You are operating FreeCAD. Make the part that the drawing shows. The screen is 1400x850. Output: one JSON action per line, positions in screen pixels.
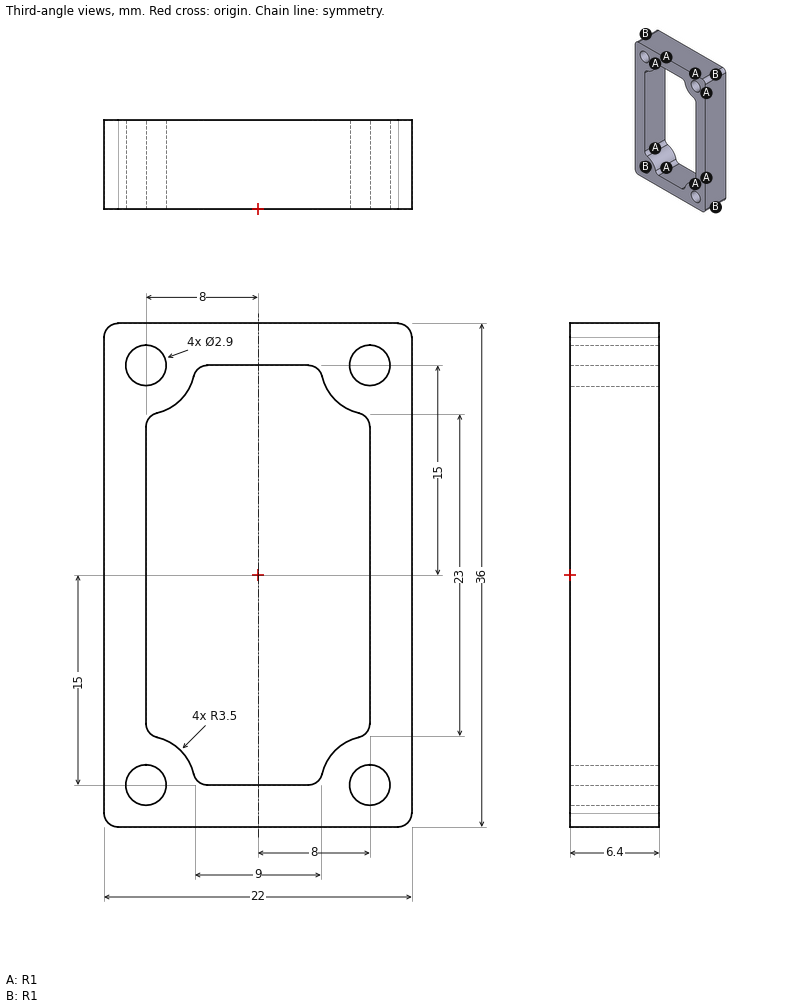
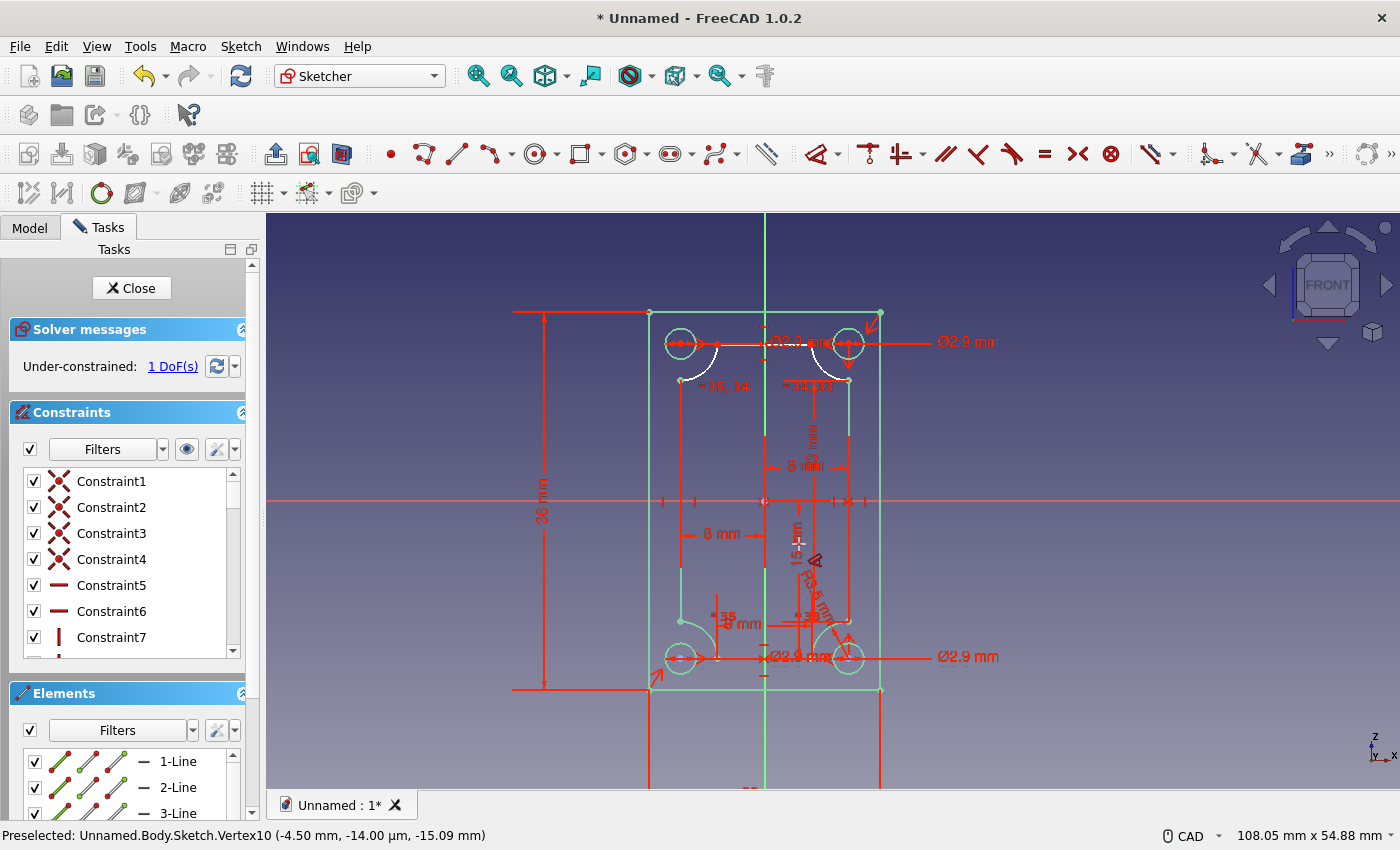
{"action": "left_click", "coordinate": [812, 345]}
{"action": "left_click", "coordinate": [731, 423]}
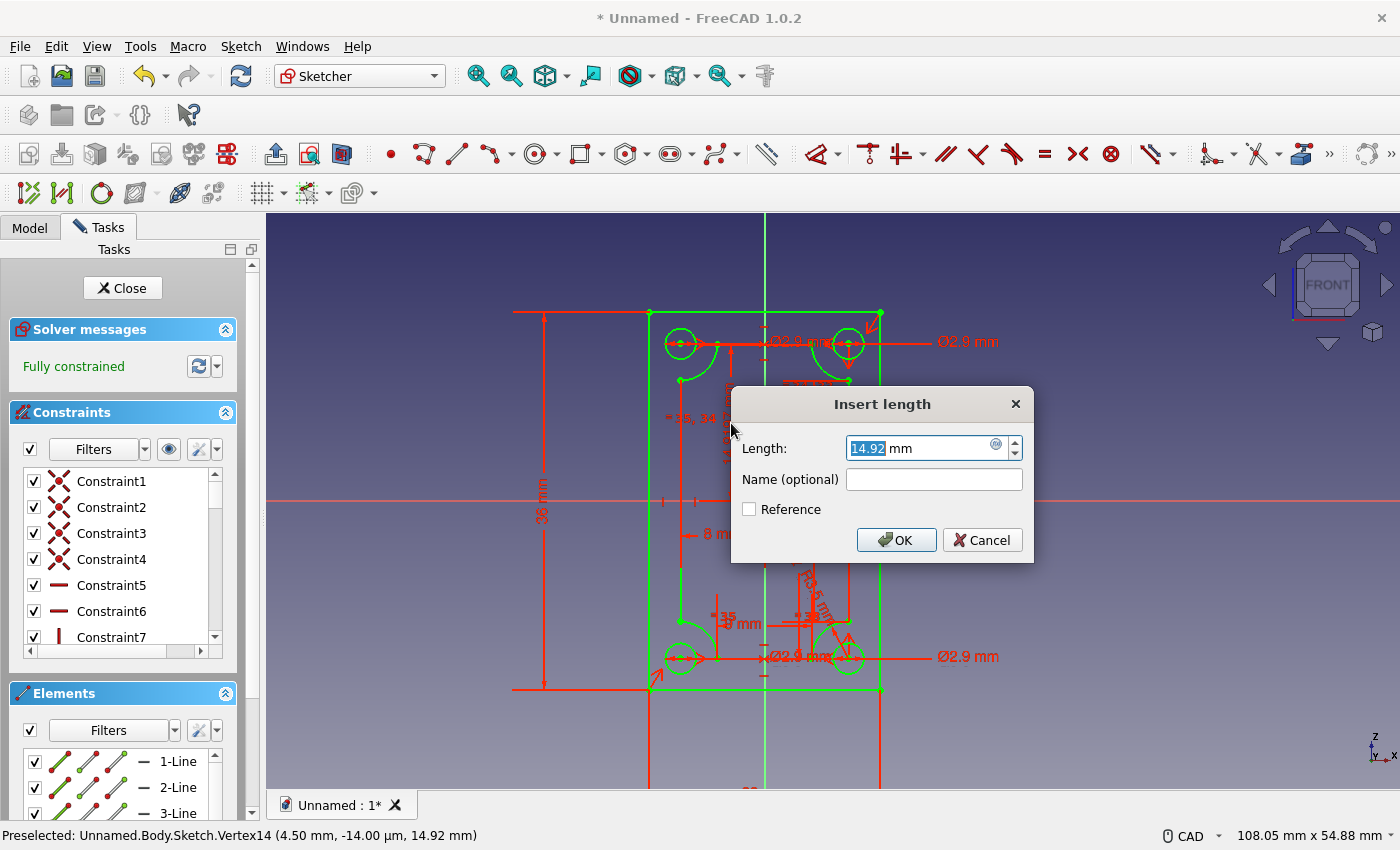
{"action": "type", "text": "15"}
{"action": "key", "text": "Return"}
{"action": "key", "text": "Escape"}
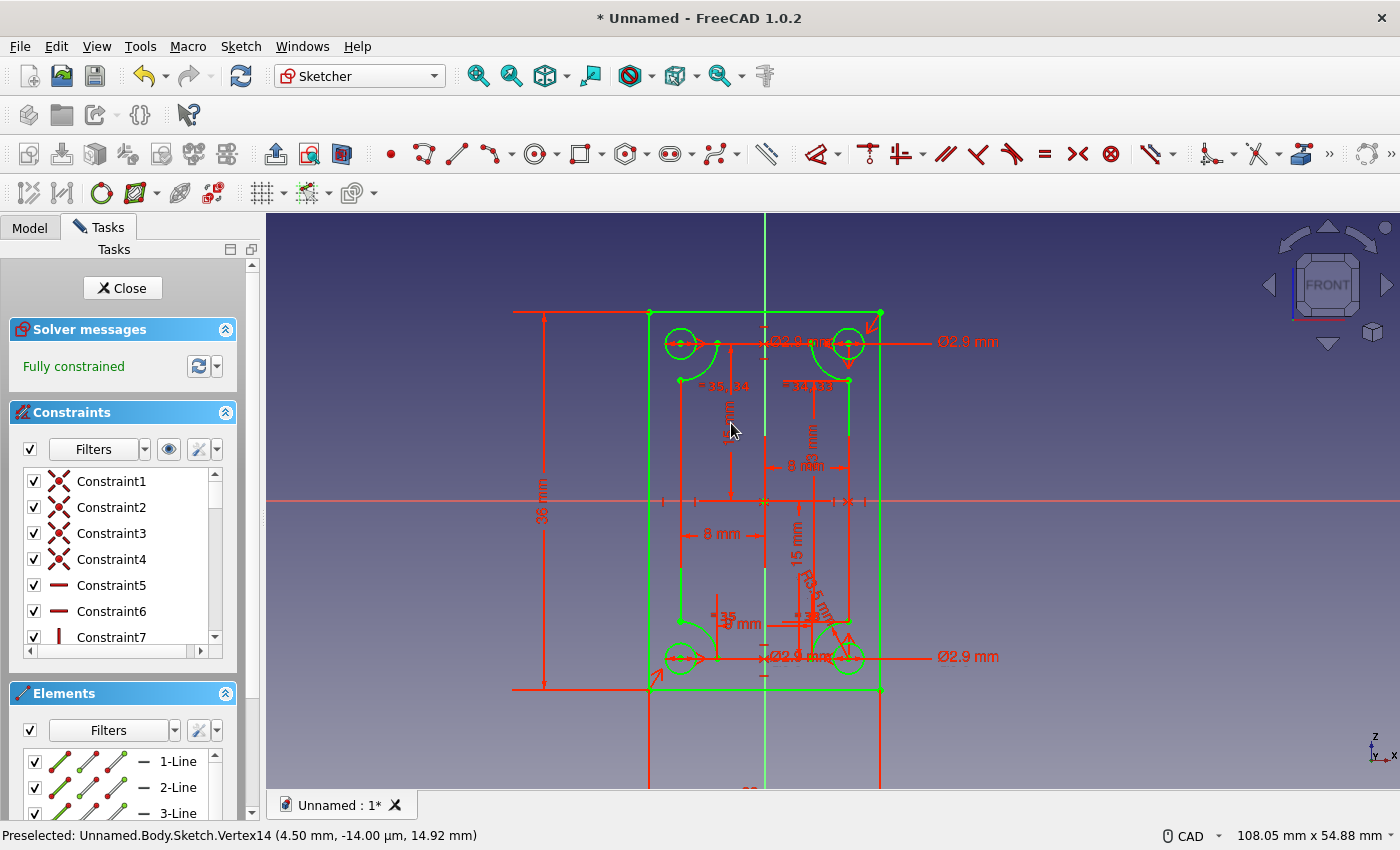
{"action": "left_click", "coordinate": [123, 288]}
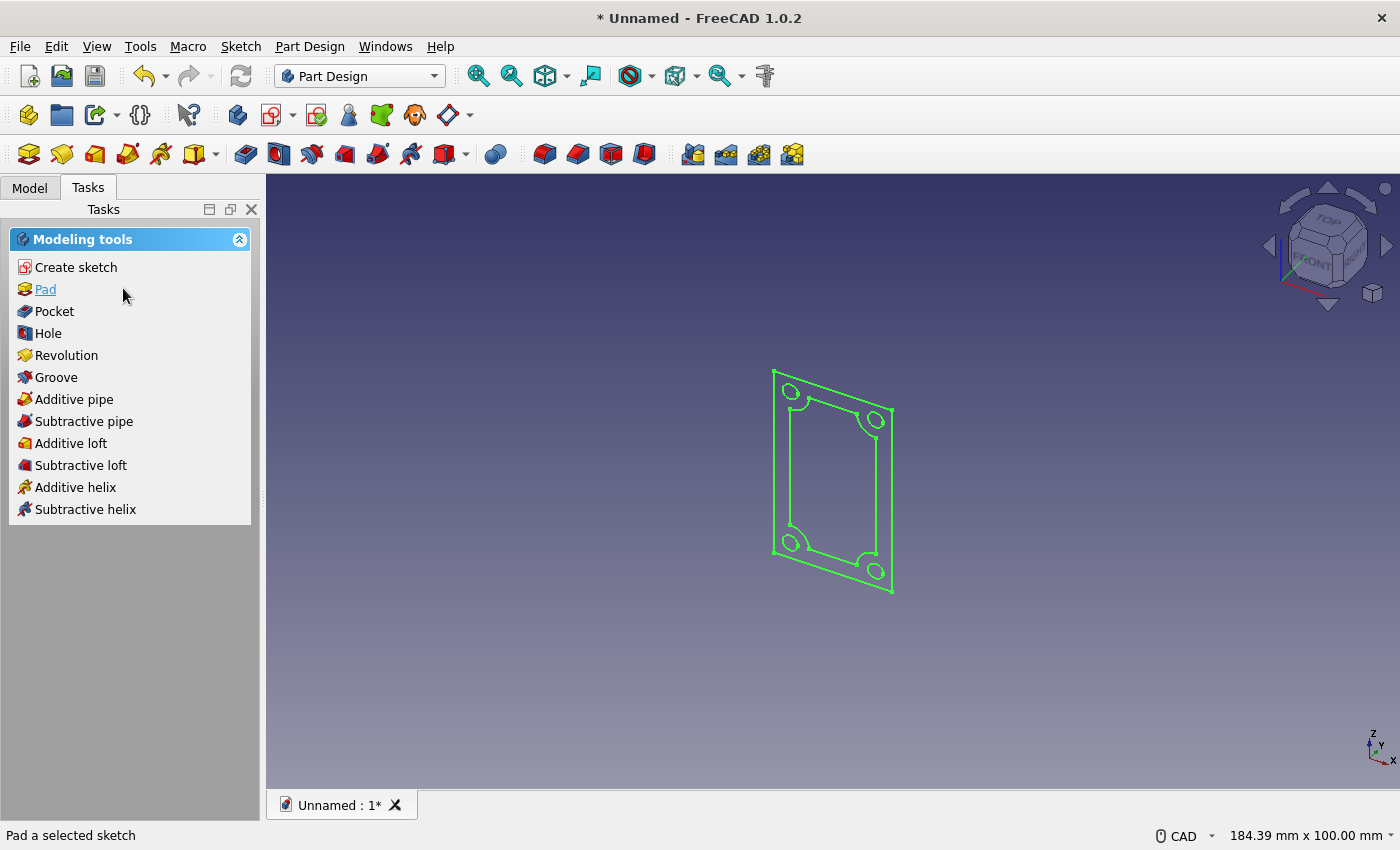
{"action": "left_click", "coordinate": [29, 154]}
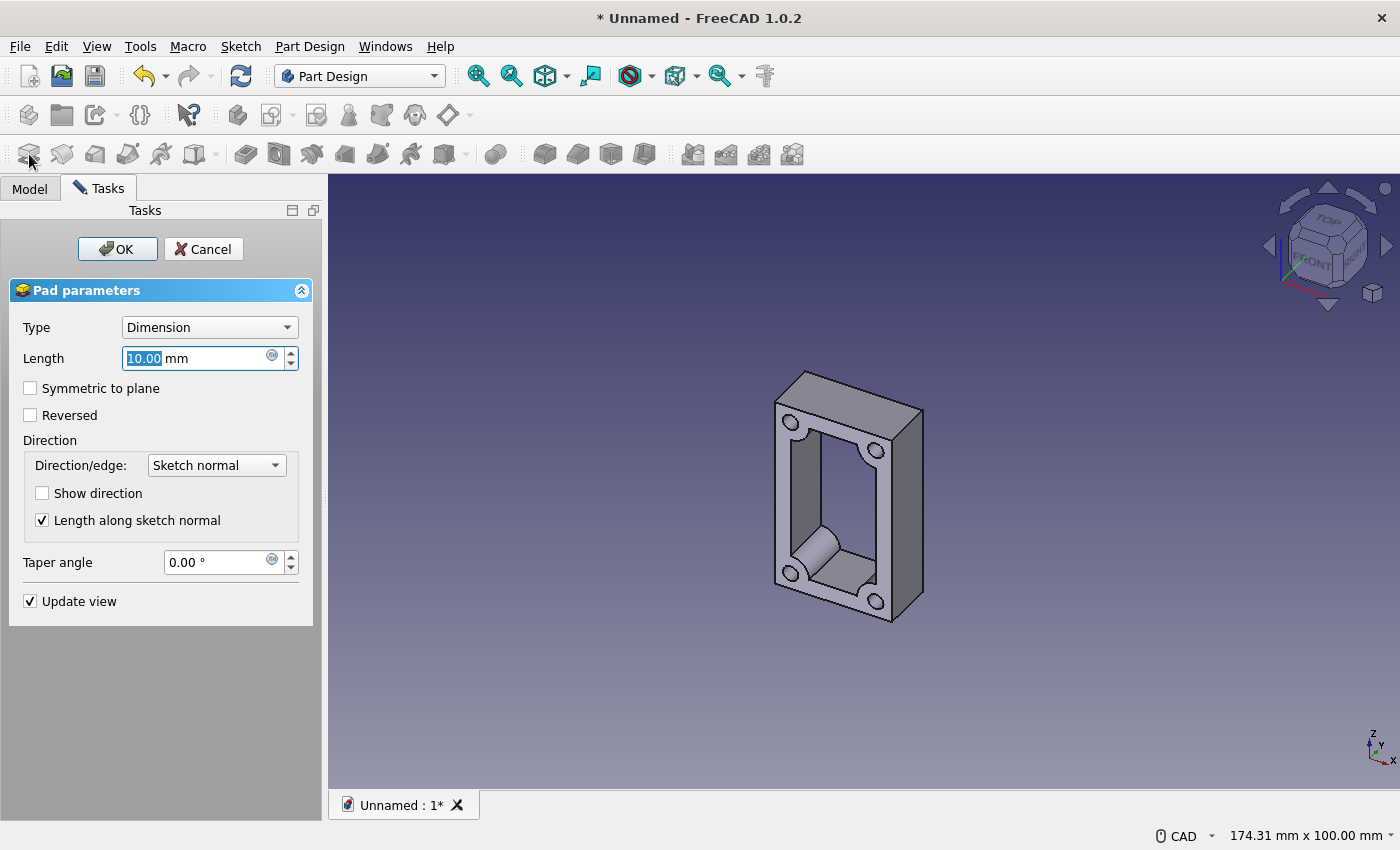
{"action": "type", "text": "6.4"}
{"action": "key", "text": "Tab"}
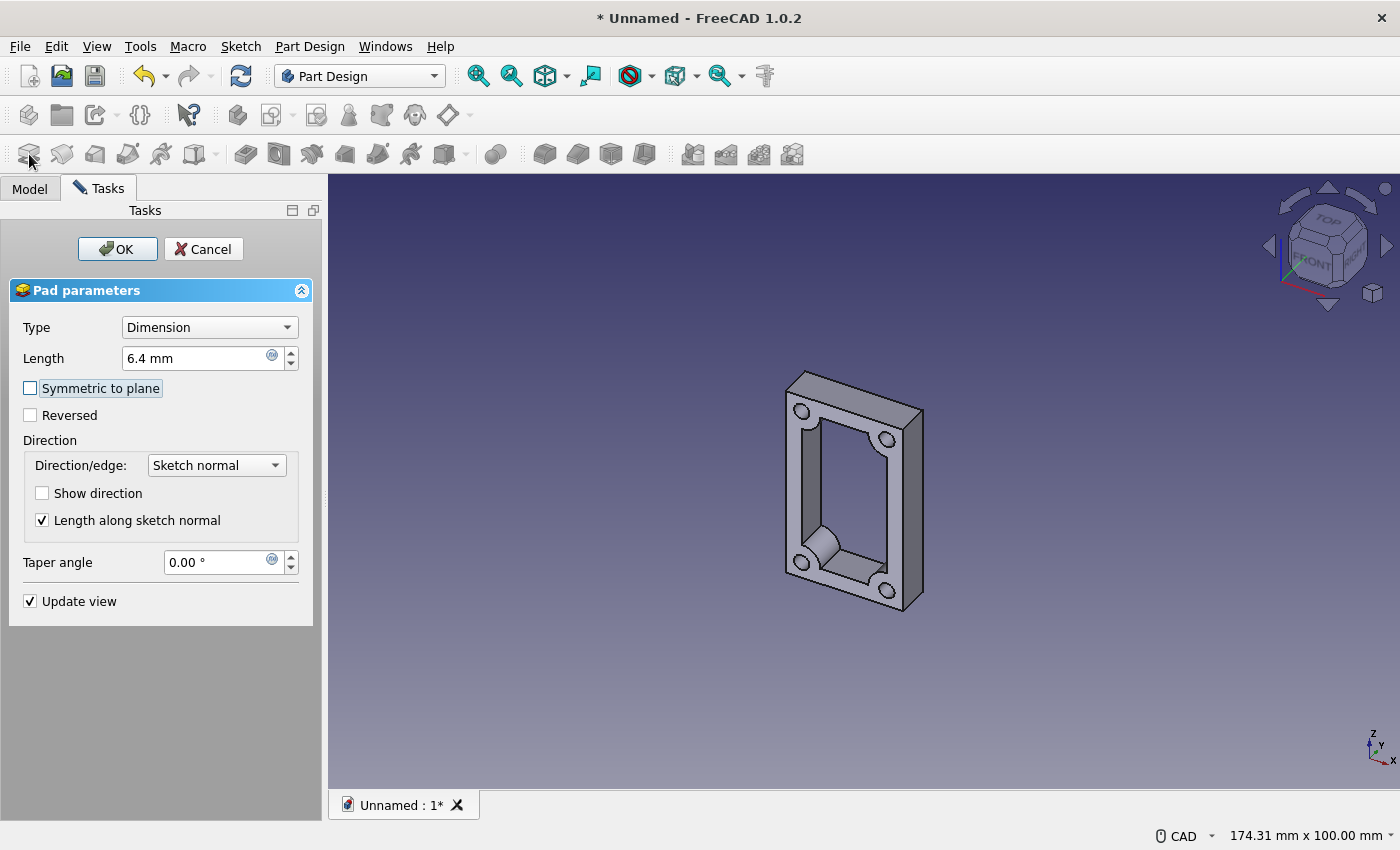
{"action": "left_click", "coordinate": [31, 415]}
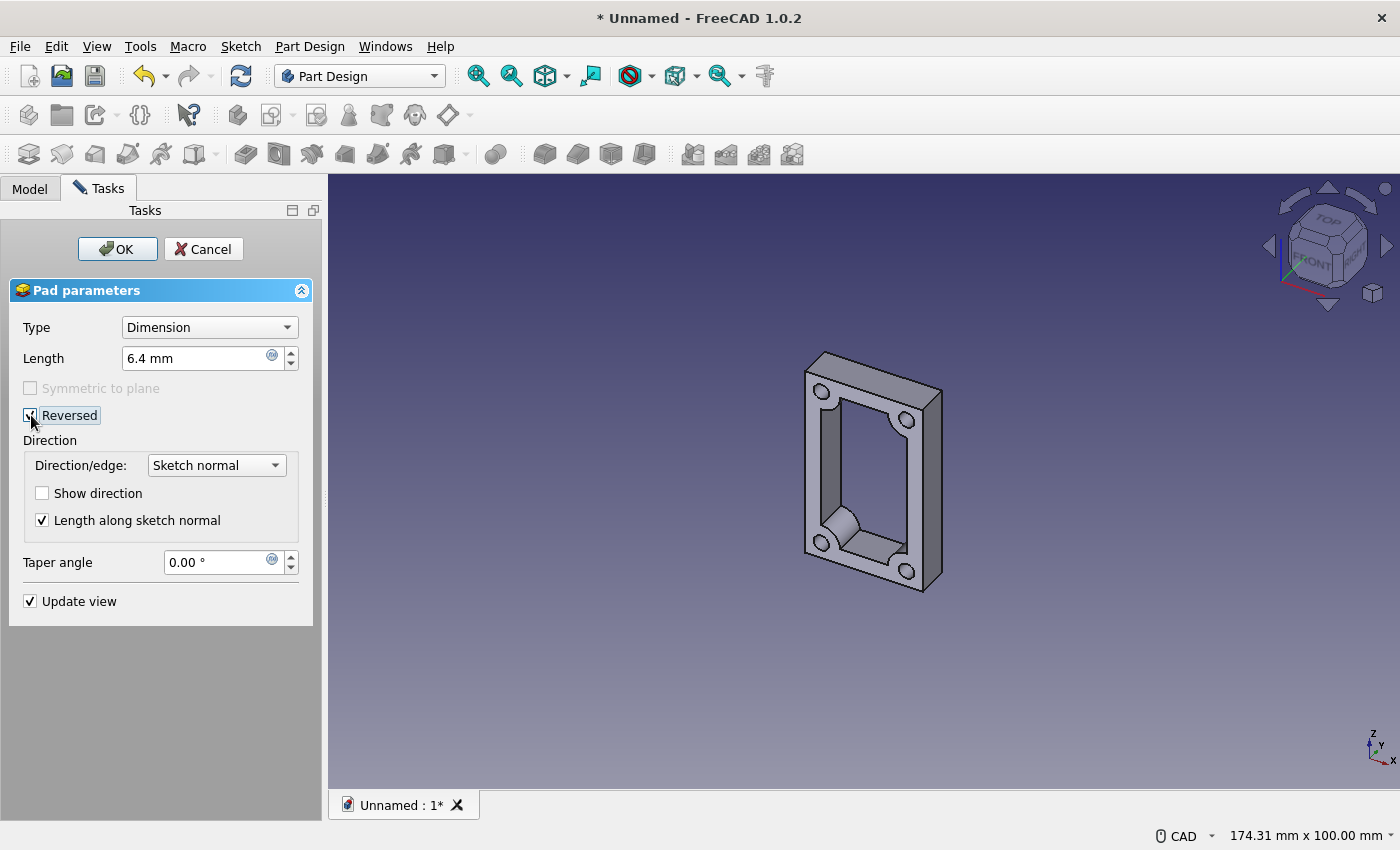
{"action": "left_click", "coordinate": [118, 249]}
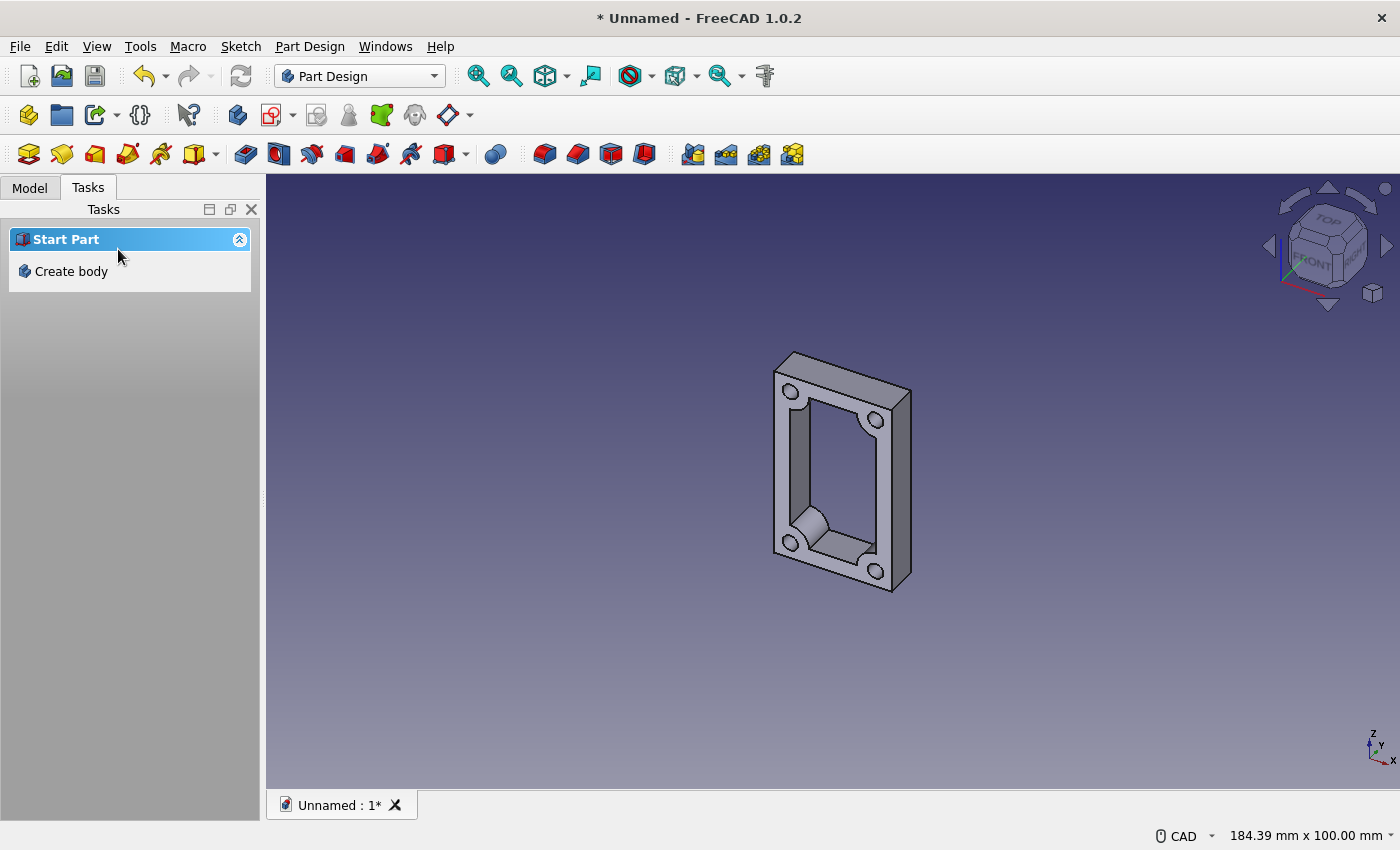
{"action": "left_click", "coordinate": [479, 76]}